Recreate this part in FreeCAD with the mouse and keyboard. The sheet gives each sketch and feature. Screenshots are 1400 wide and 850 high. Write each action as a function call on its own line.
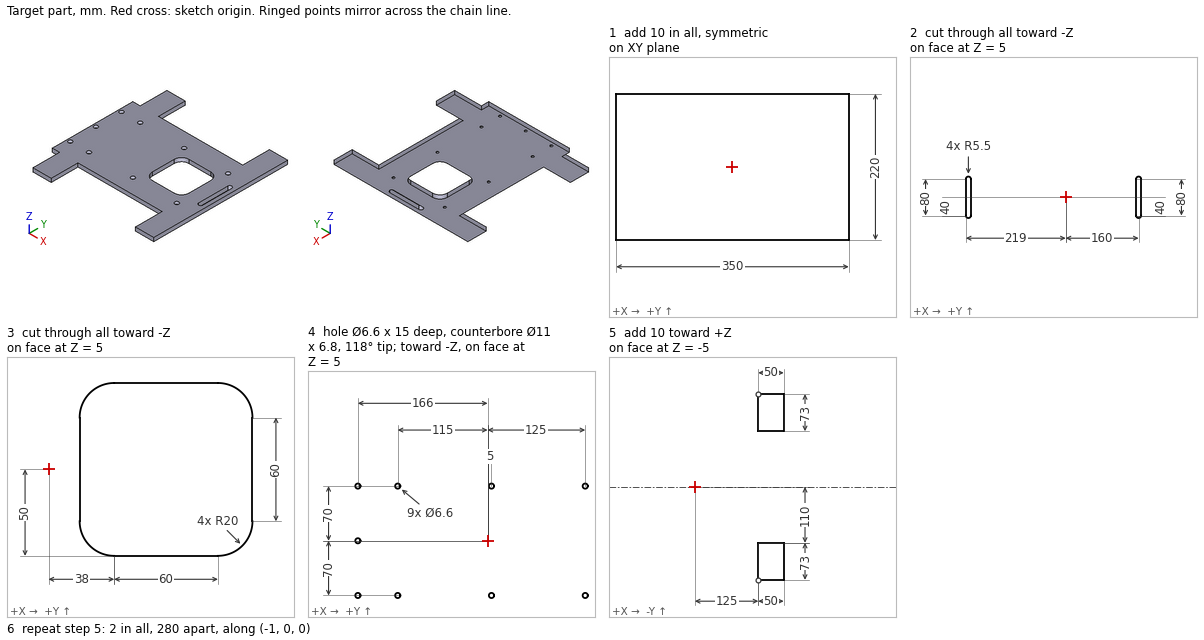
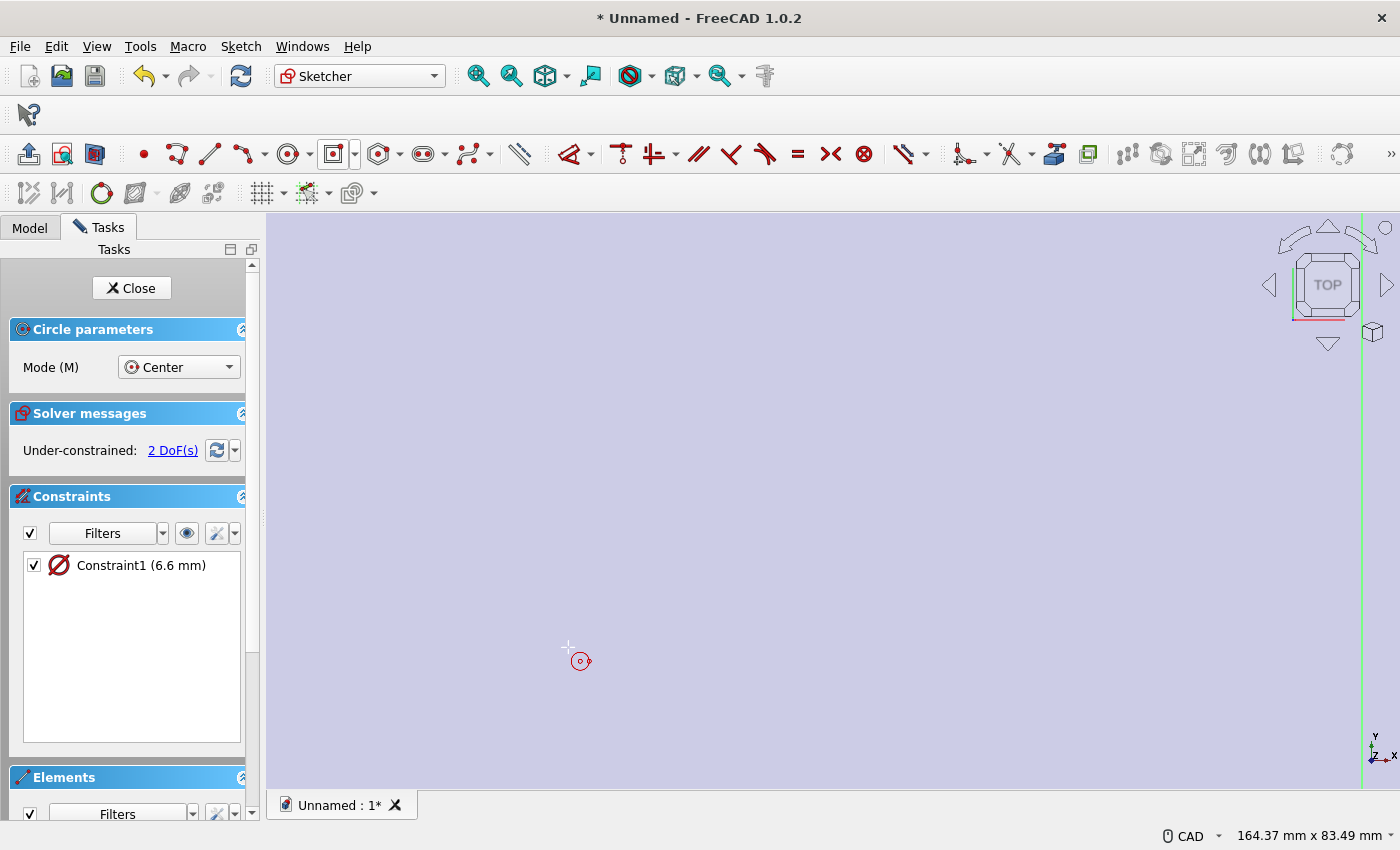
click(569, 645)
move(585, 629)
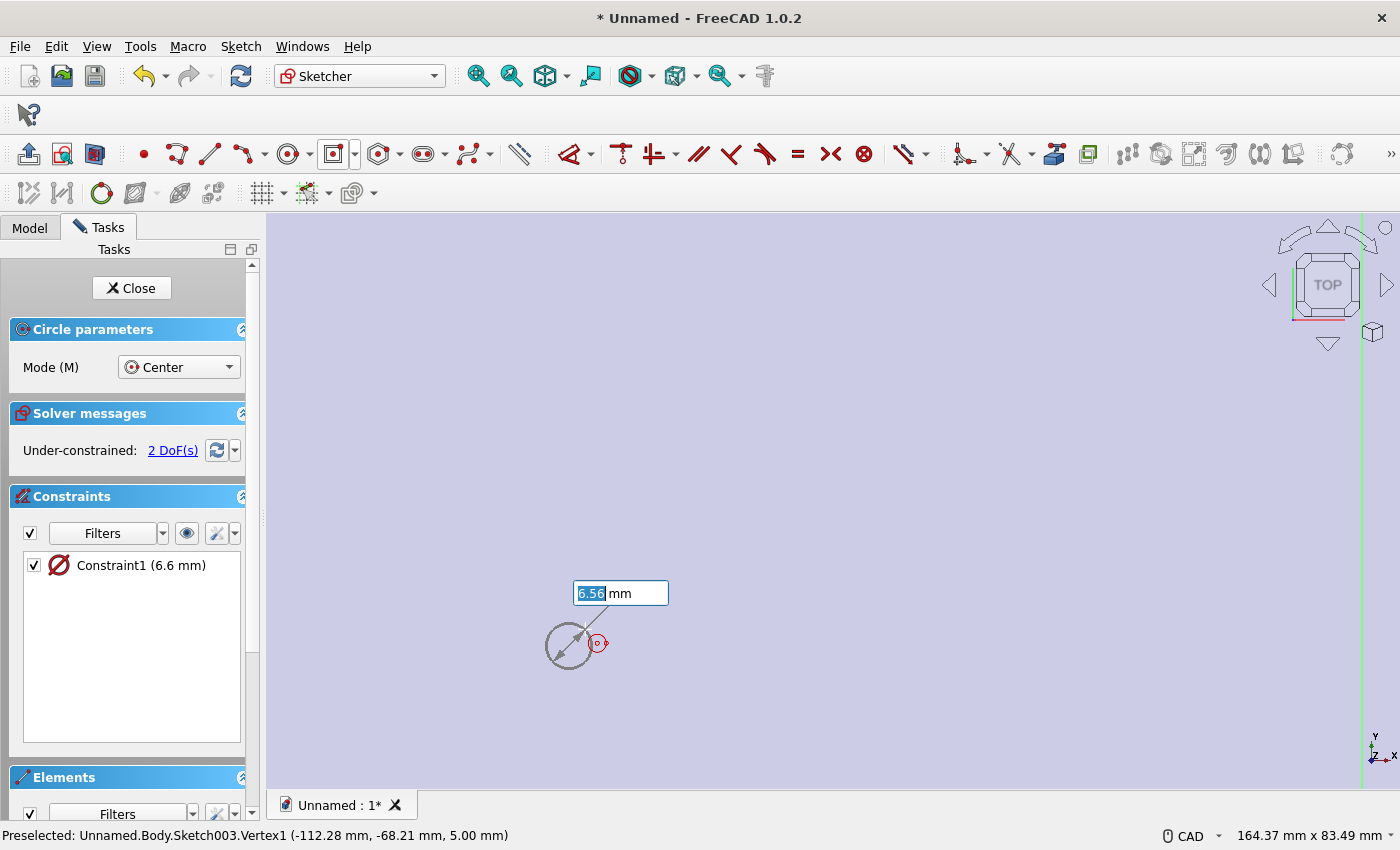
text(6.6)
key(Return)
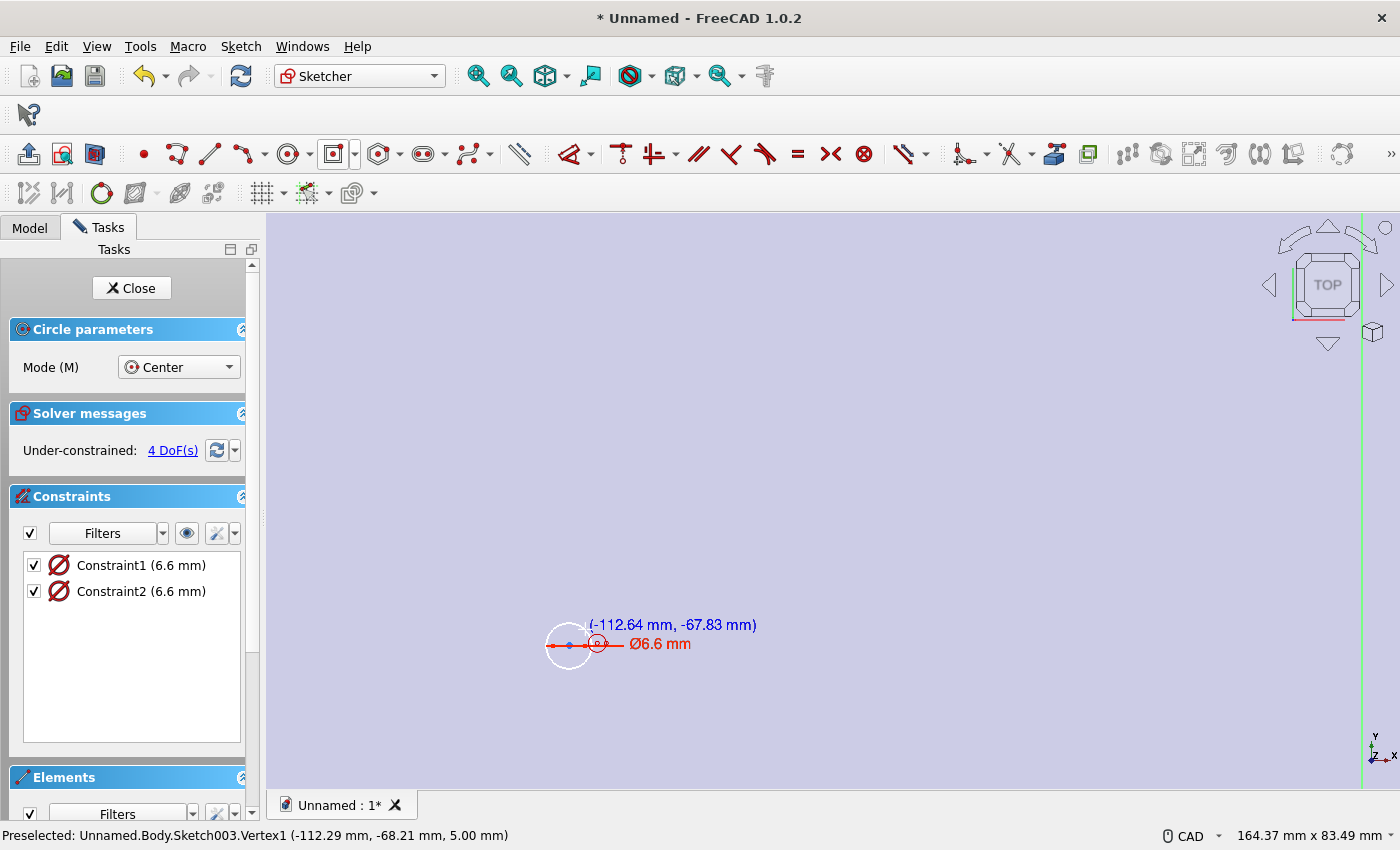
scroll(568, 647, down, 6)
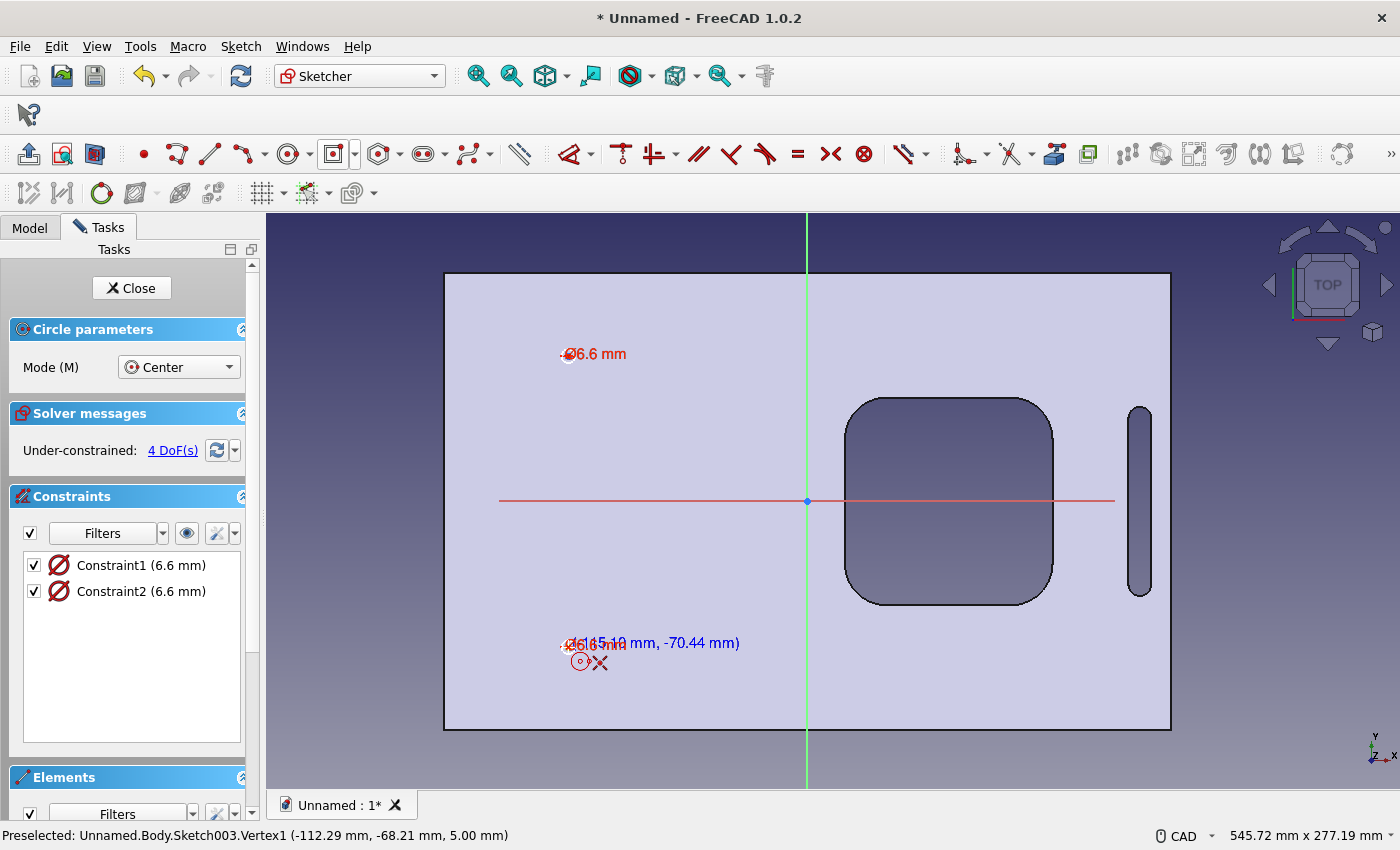
scroll(462, 356, up, 6)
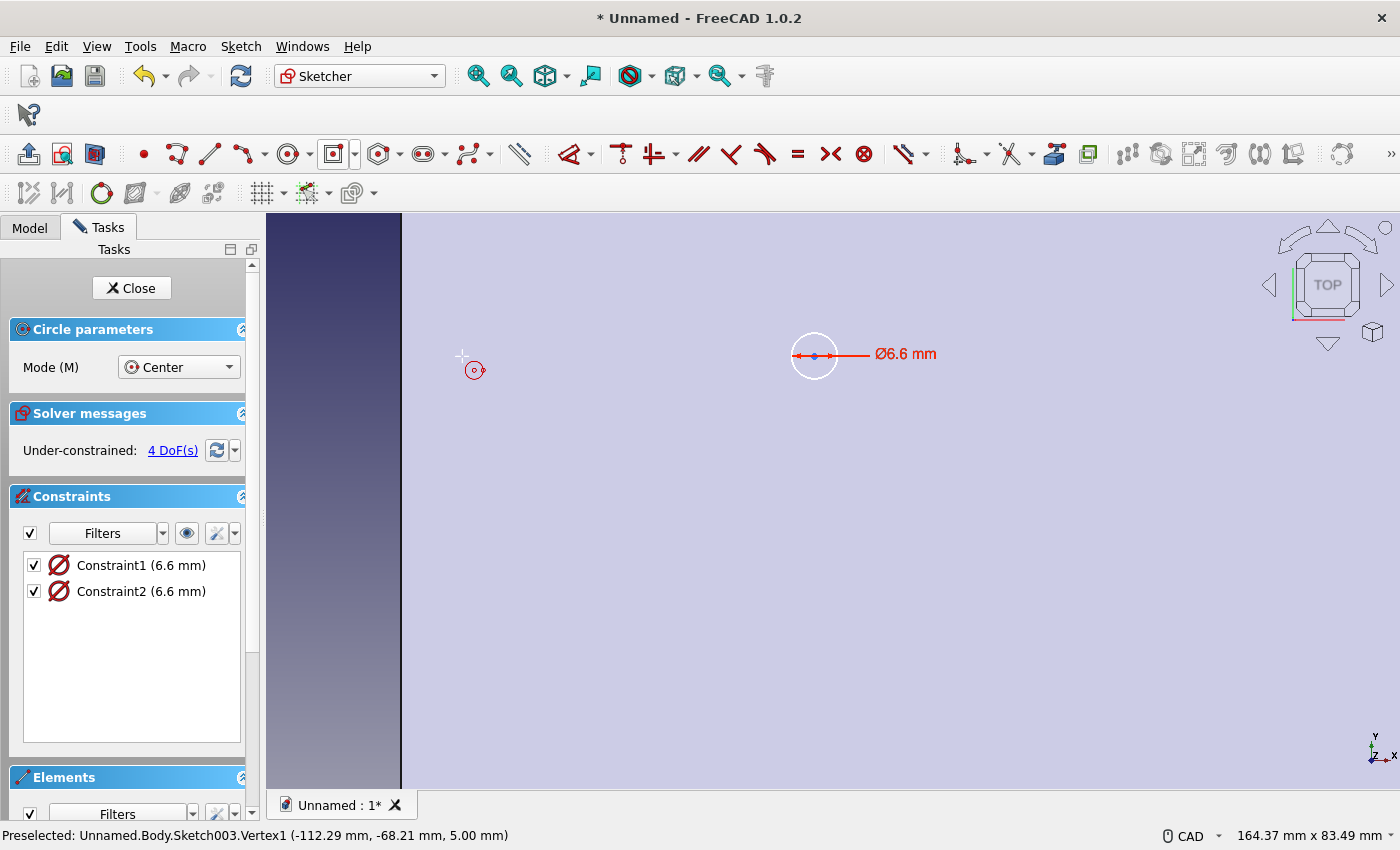
click(463, 355)
move(479, 339)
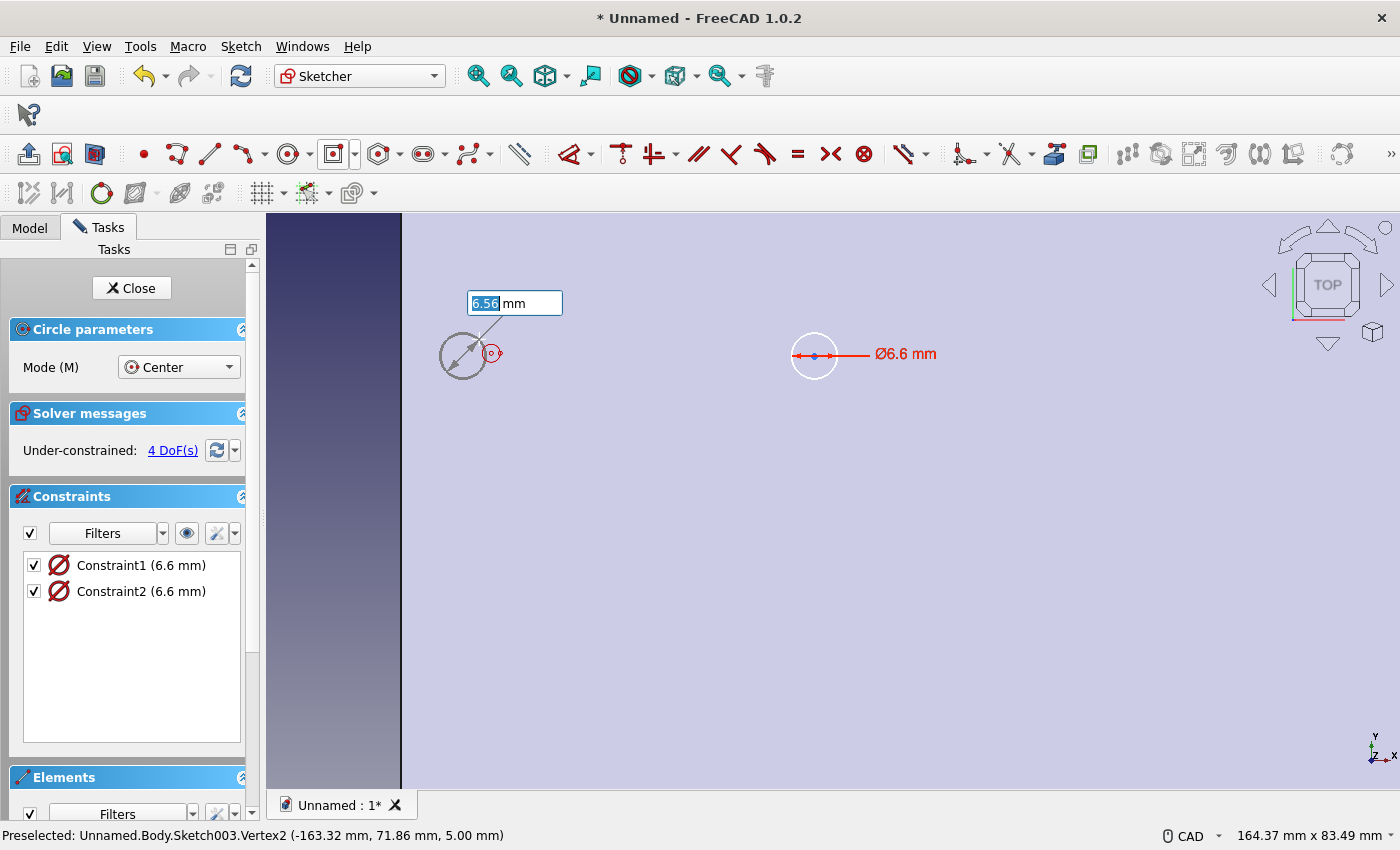
text(6.6)
key(Return)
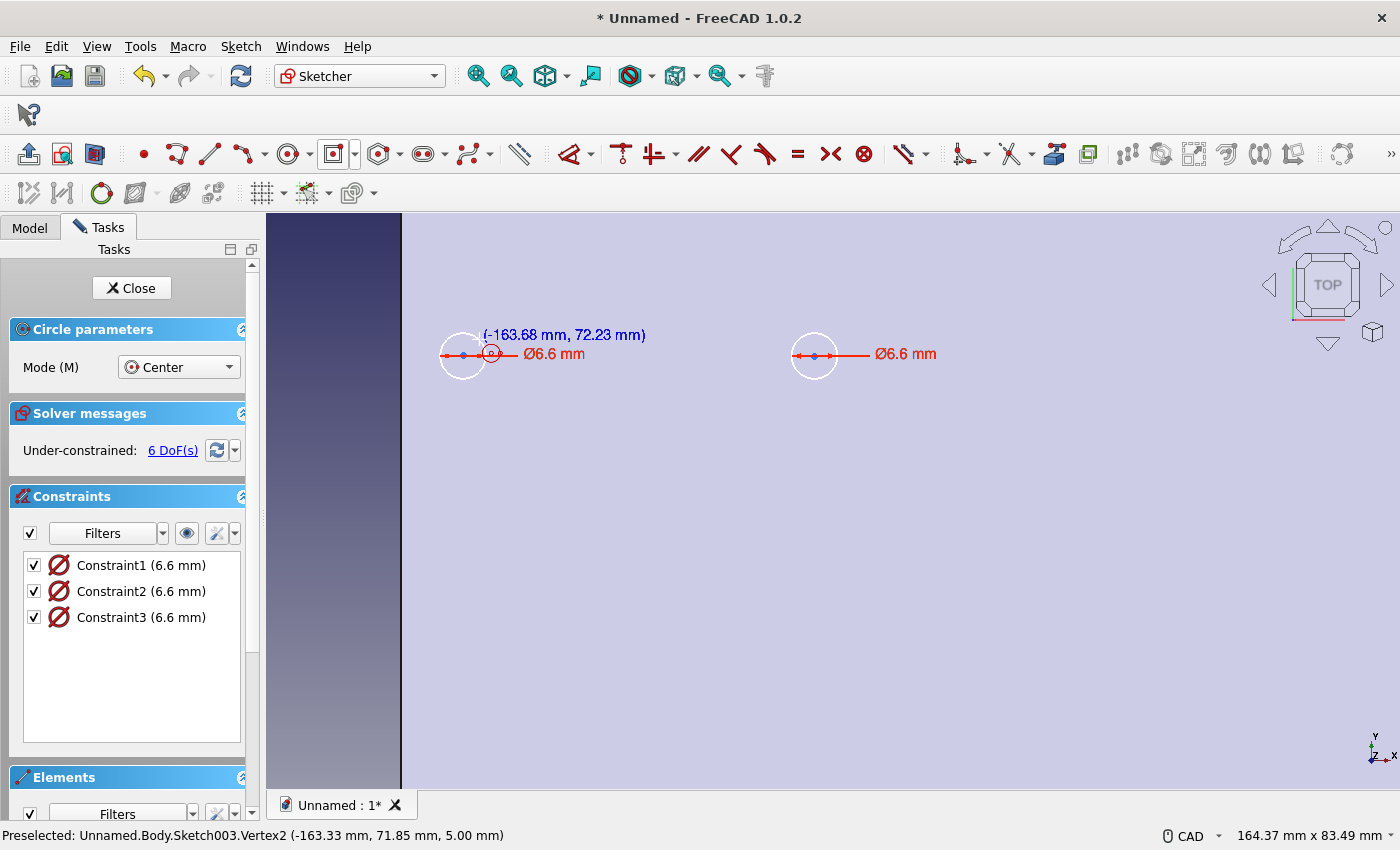
scroll(462, 356, down, 6)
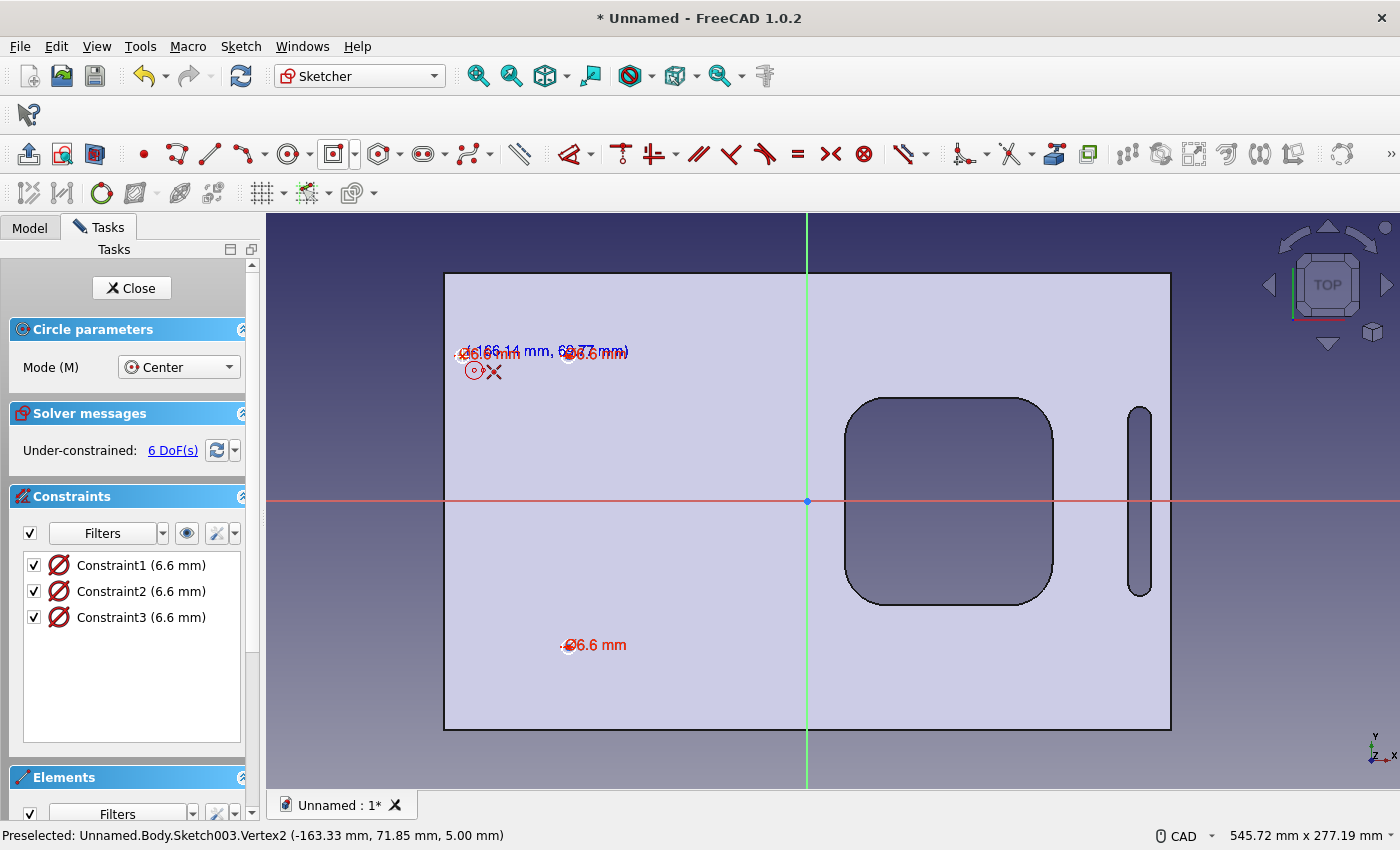
scroll(462, 647, up, 6)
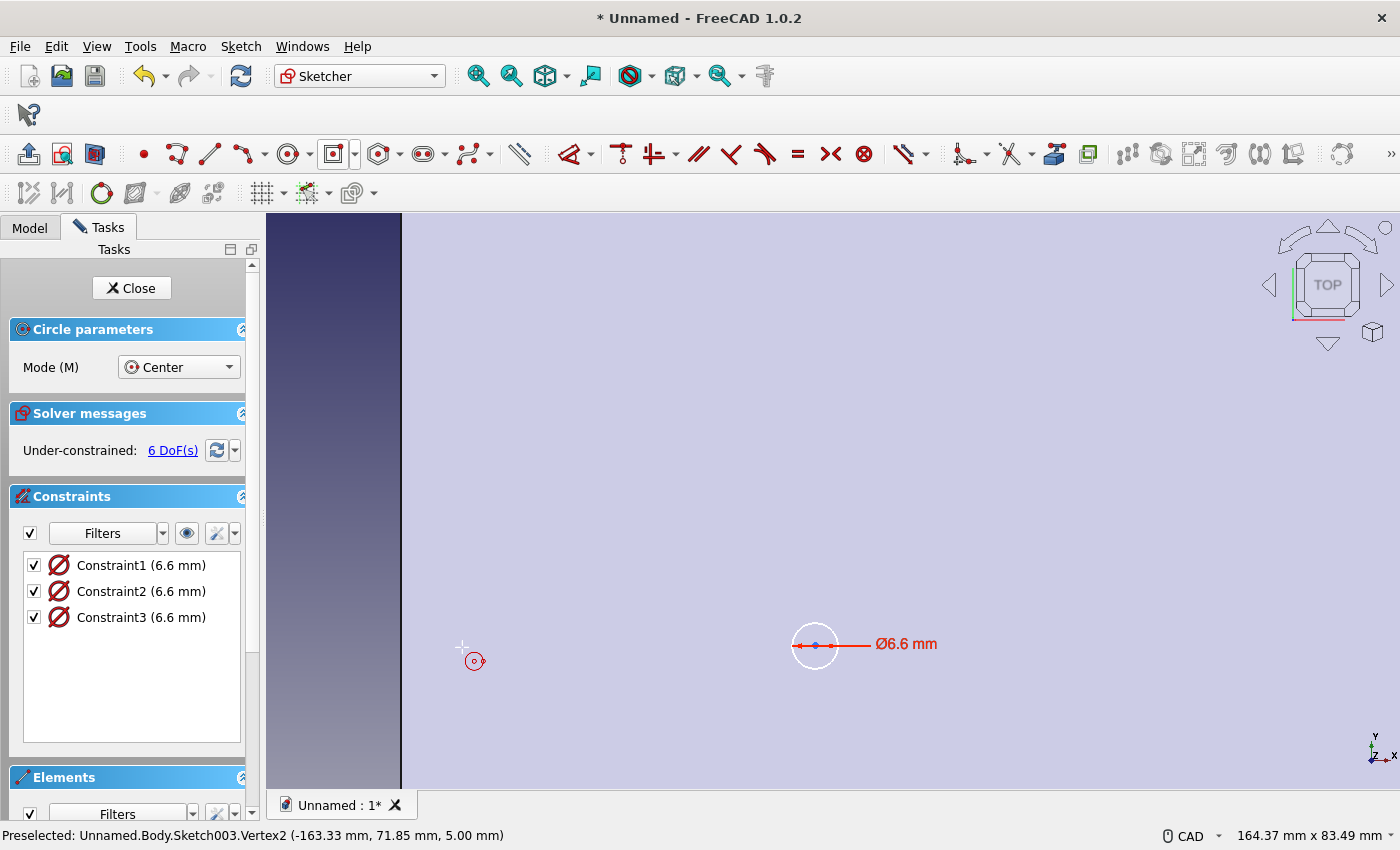
click(463, 645)
move(479, 629)